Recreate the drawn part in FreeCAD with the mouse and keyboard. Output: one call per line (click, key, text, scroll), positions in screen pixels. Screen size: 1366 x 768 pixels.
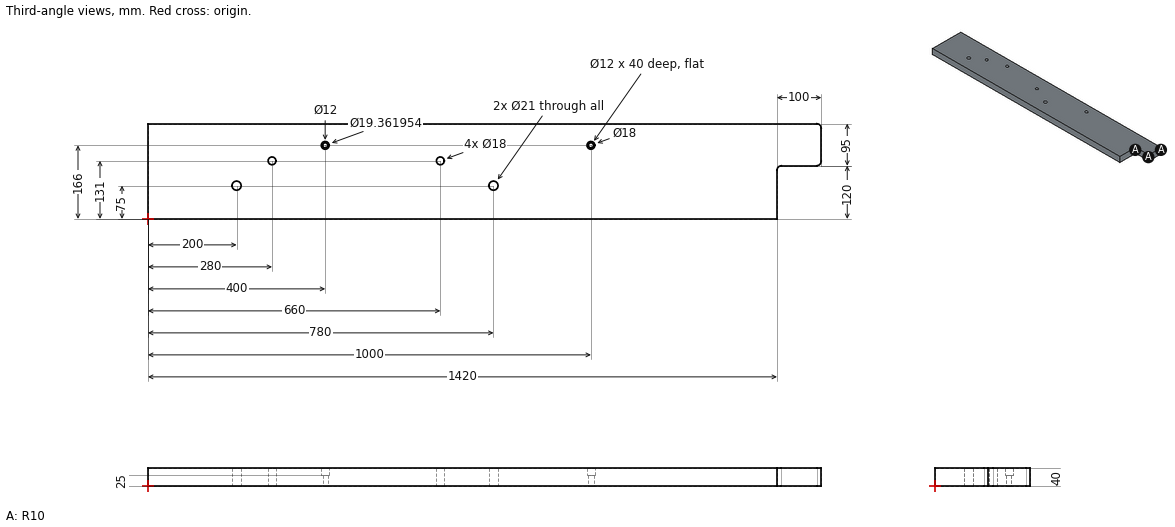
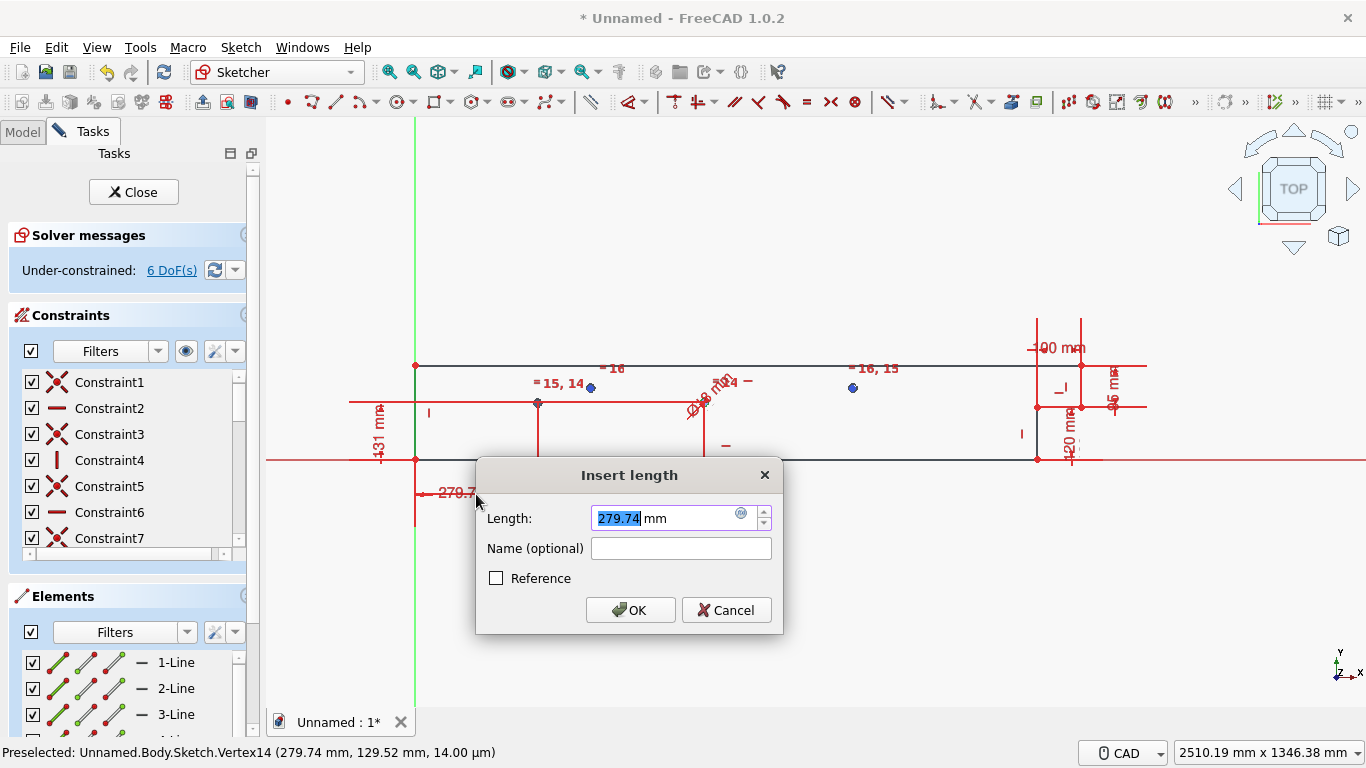
text(280)
key(Return)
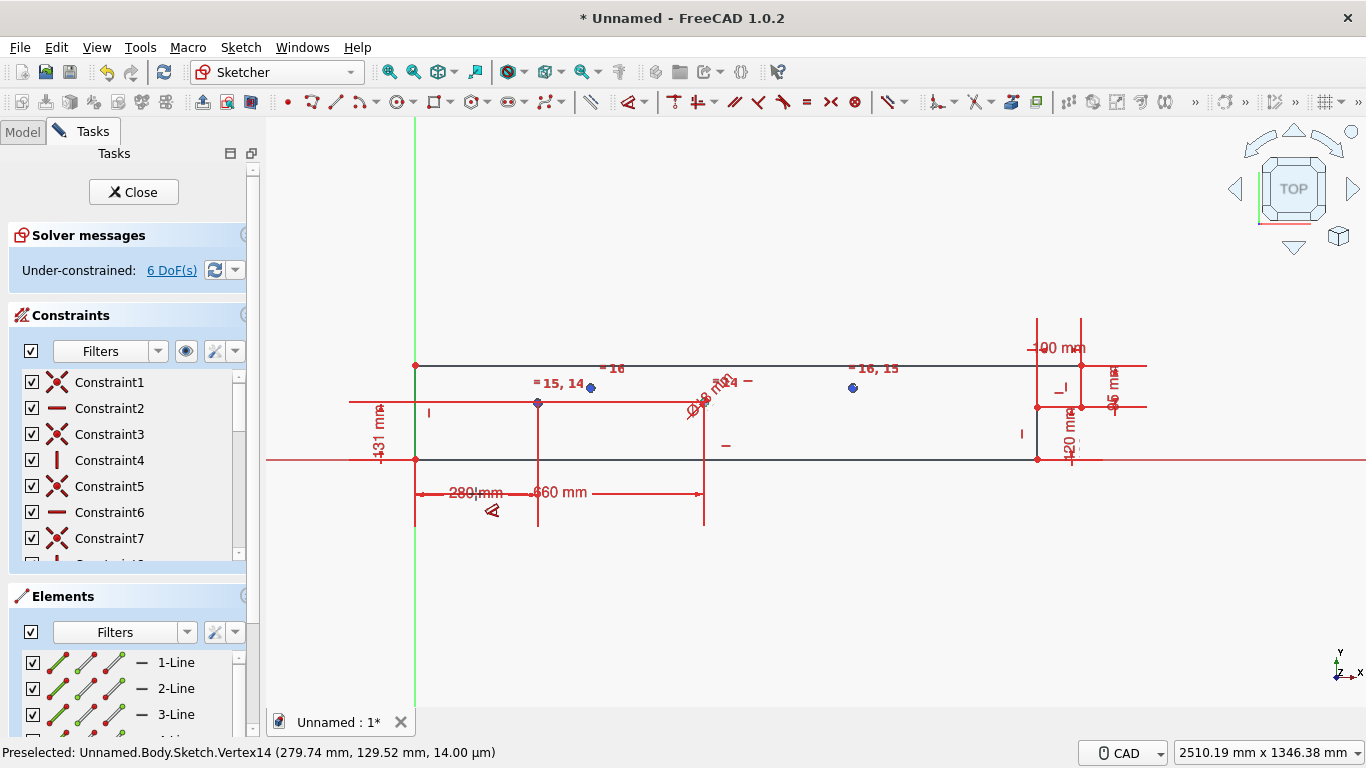
click(538, 403)
click(572, 431)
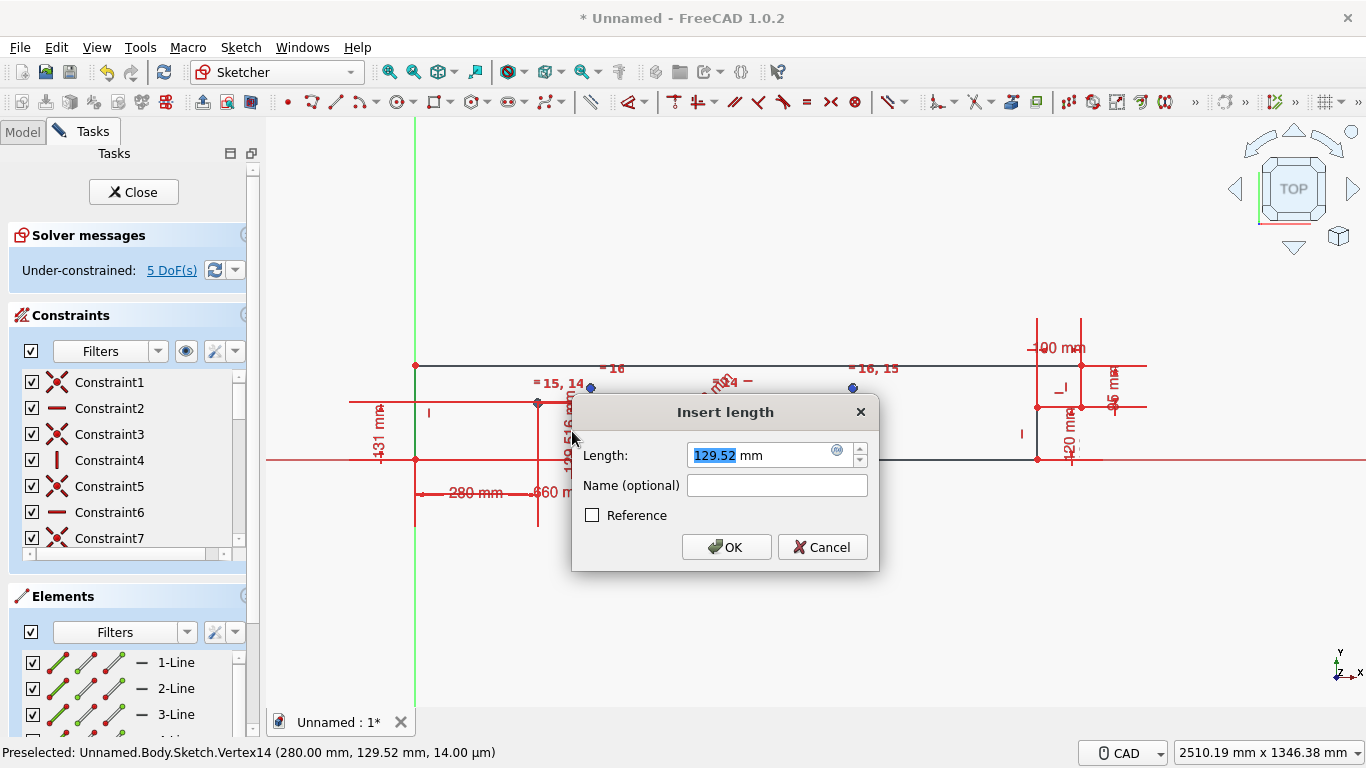
text(131)
key(Return)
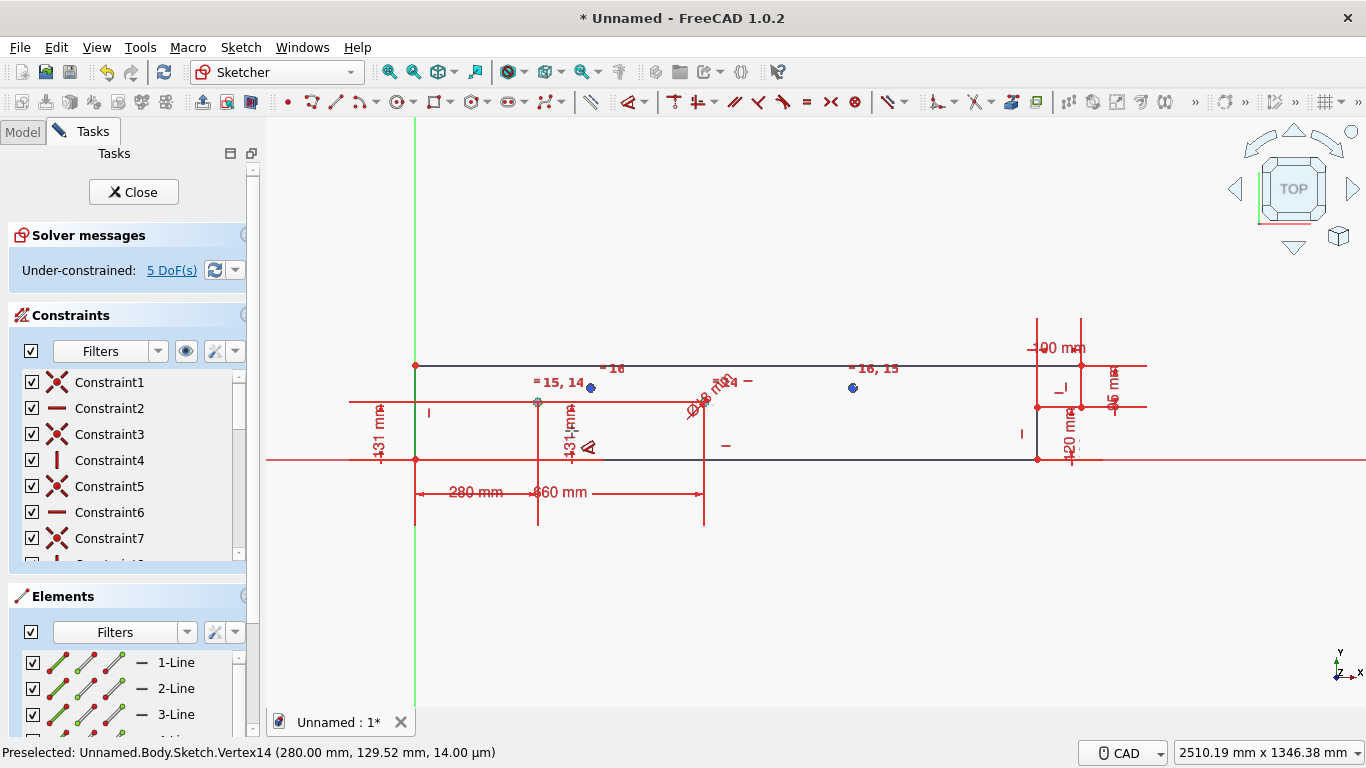
click(853, 388)
click(381, 407)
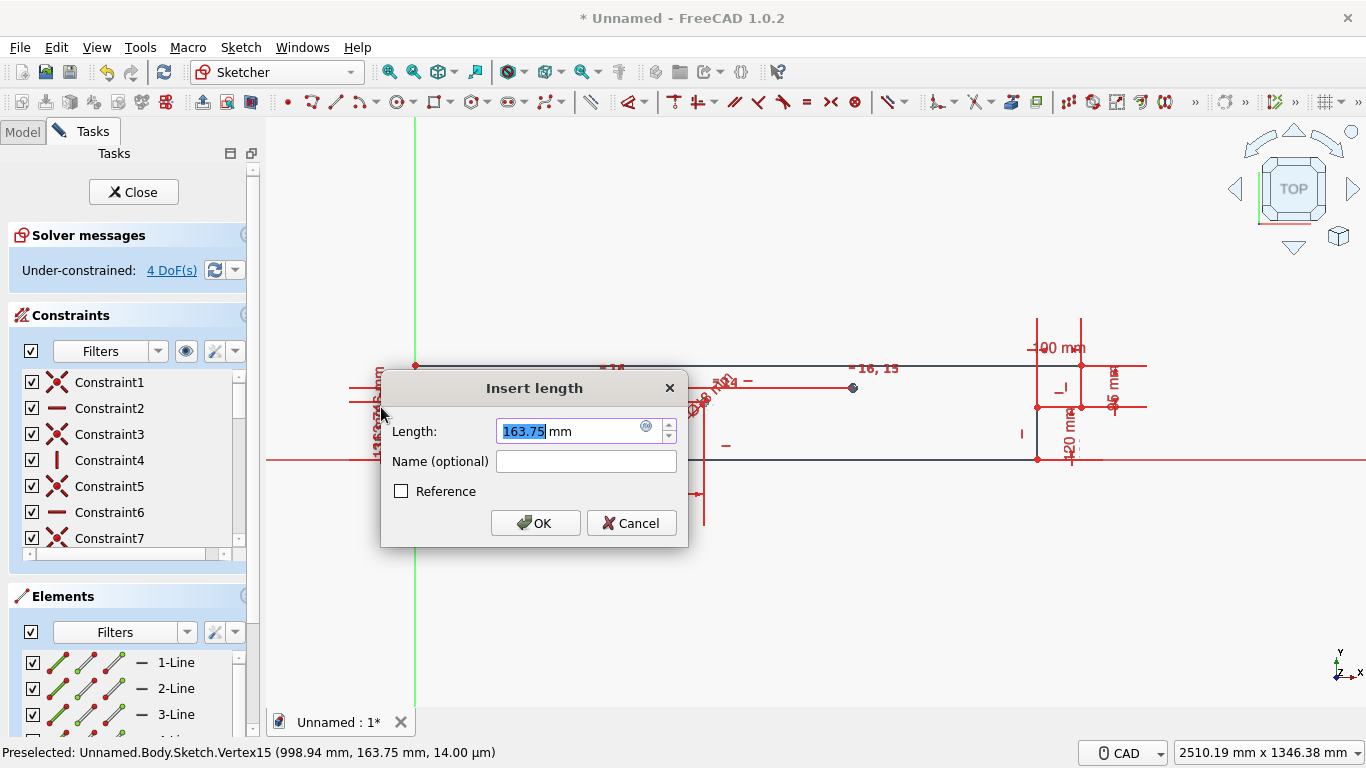
text(166)
key(Return)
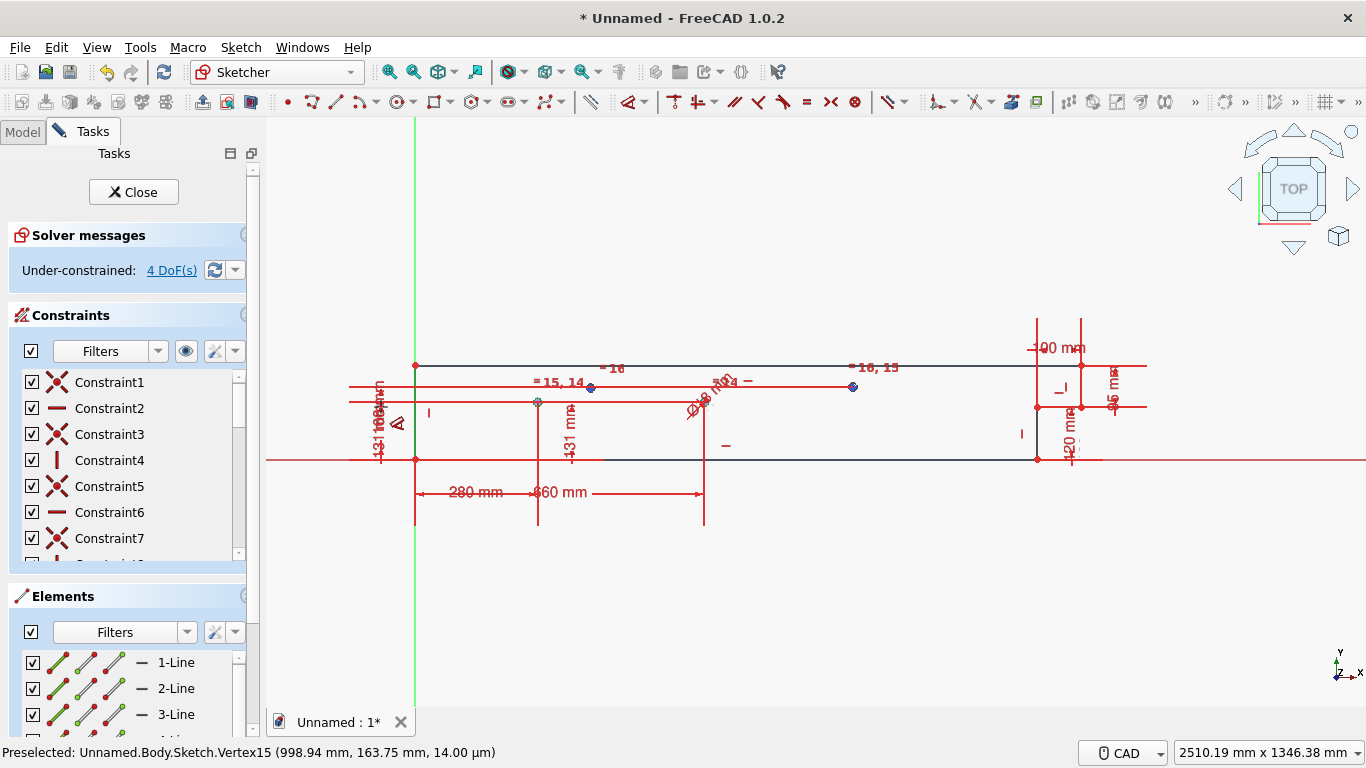
click(591, 388)
click(503, 518)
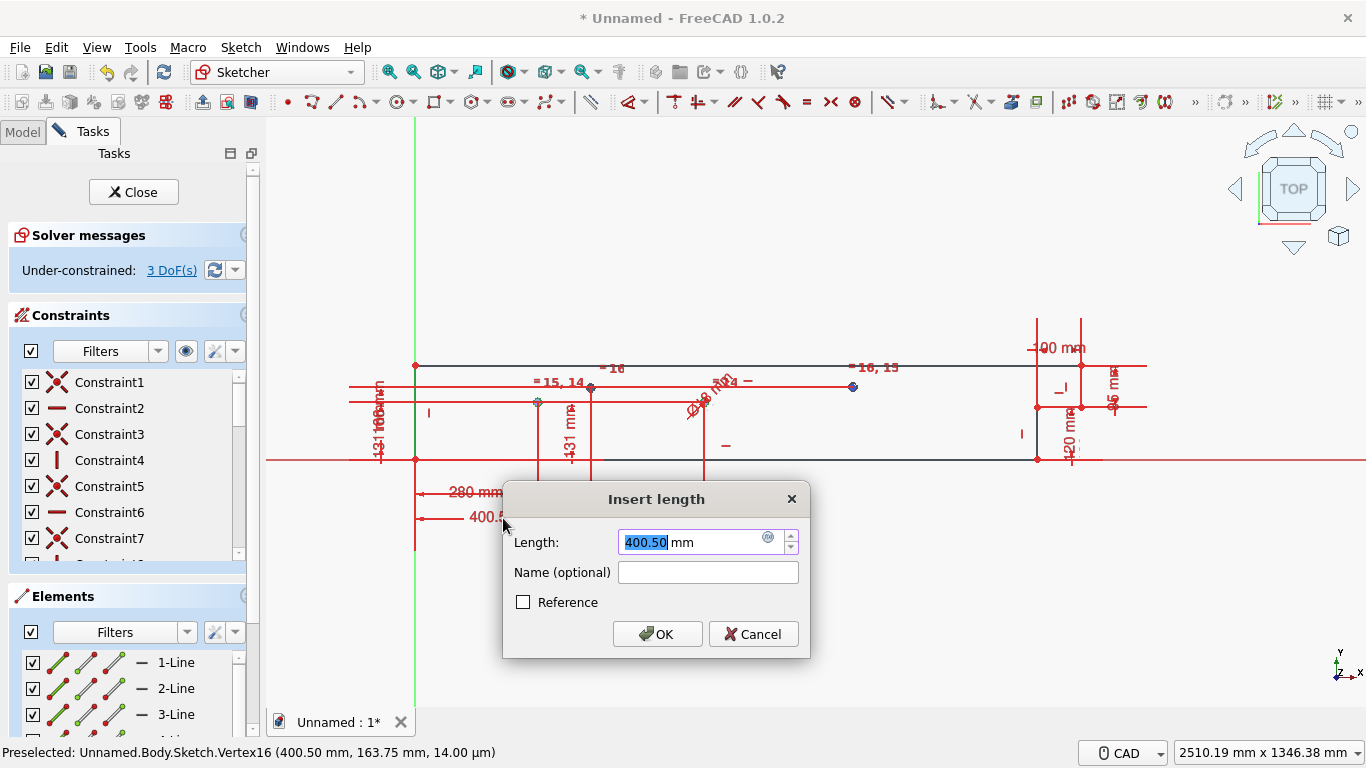
text(400)
key(Return)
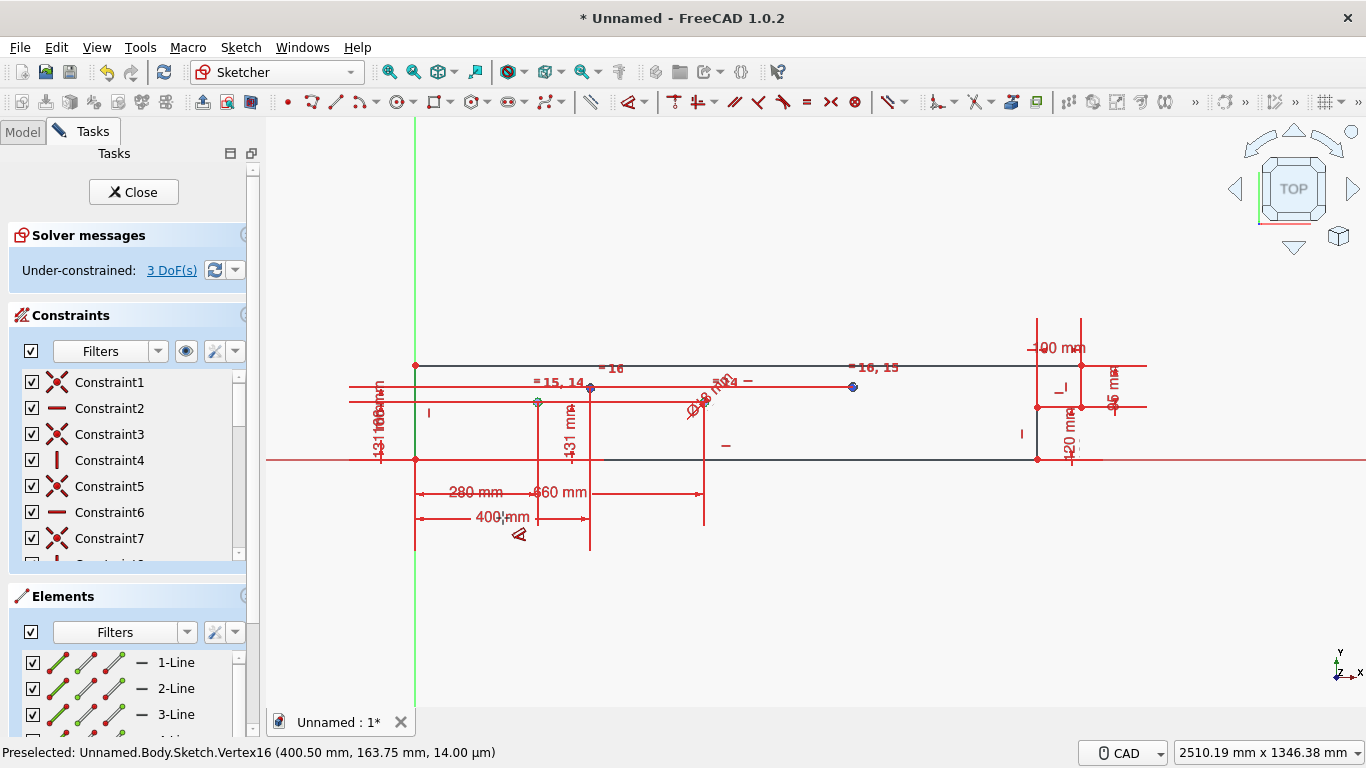
click(590, 388)
click(624, 407)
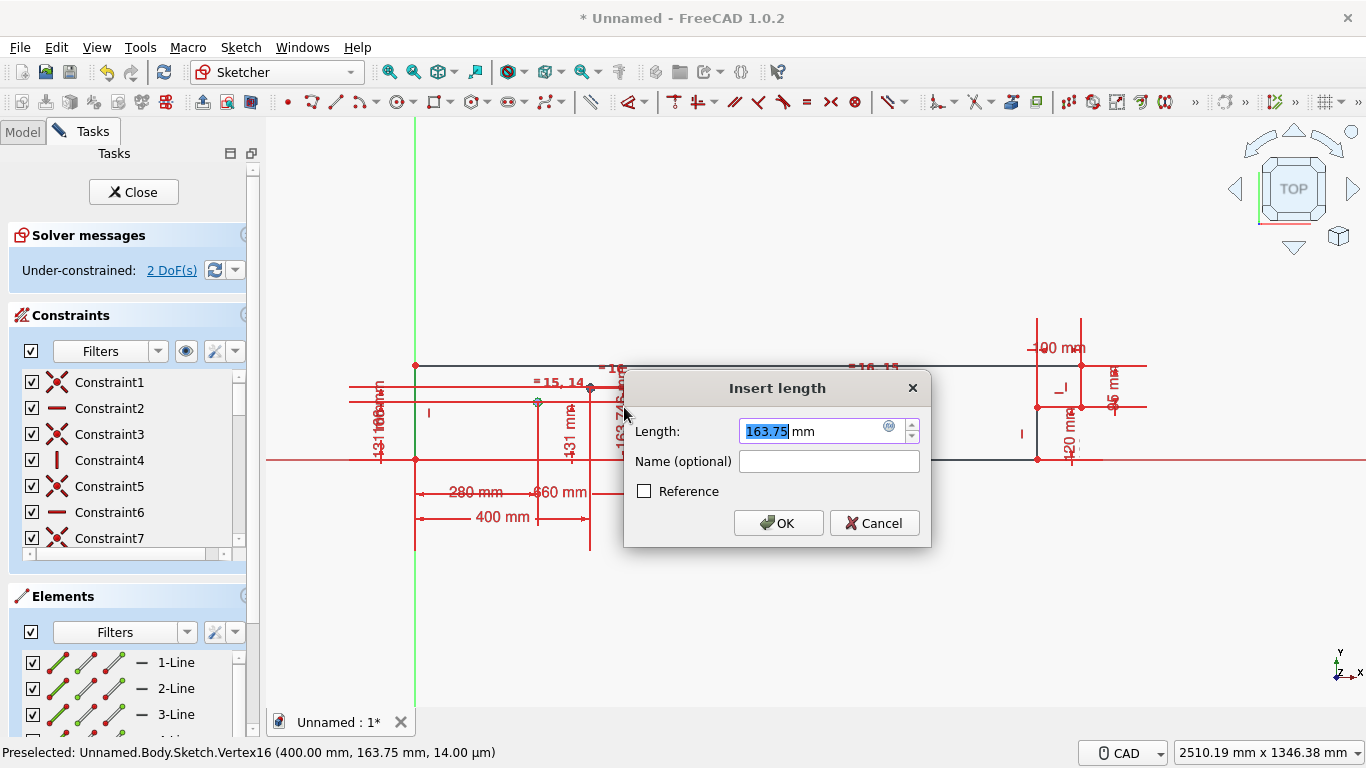
text(166)
key(Return)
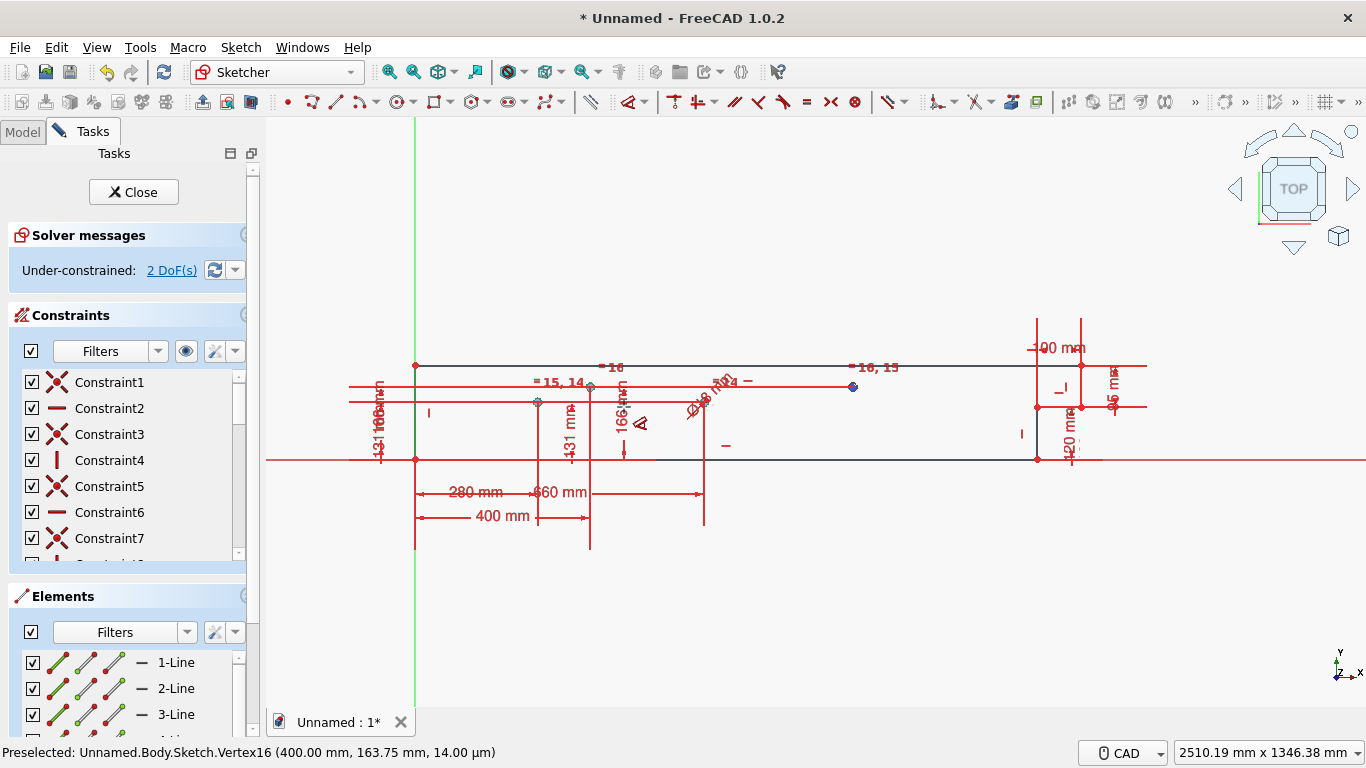
click(602, 460)
click(726, 494)